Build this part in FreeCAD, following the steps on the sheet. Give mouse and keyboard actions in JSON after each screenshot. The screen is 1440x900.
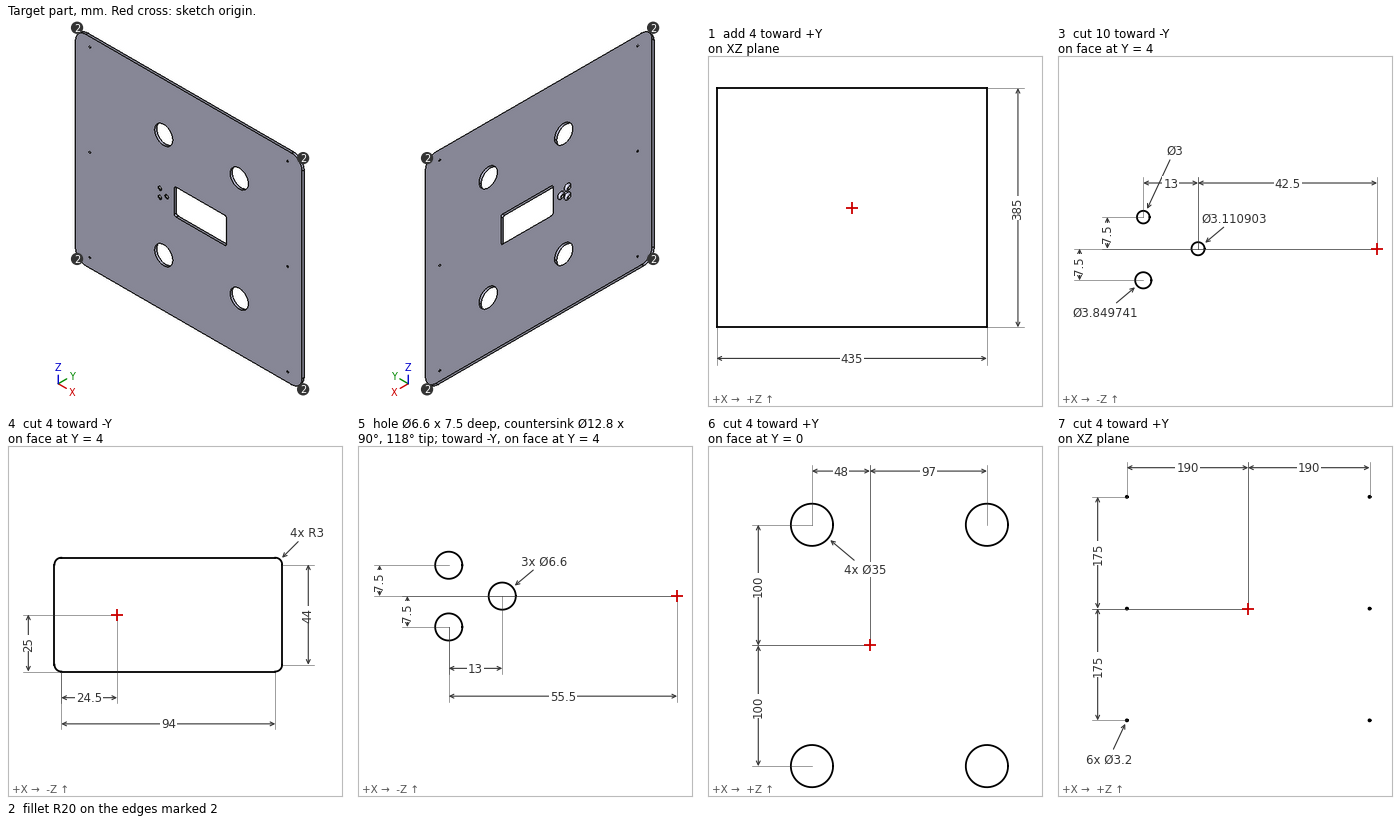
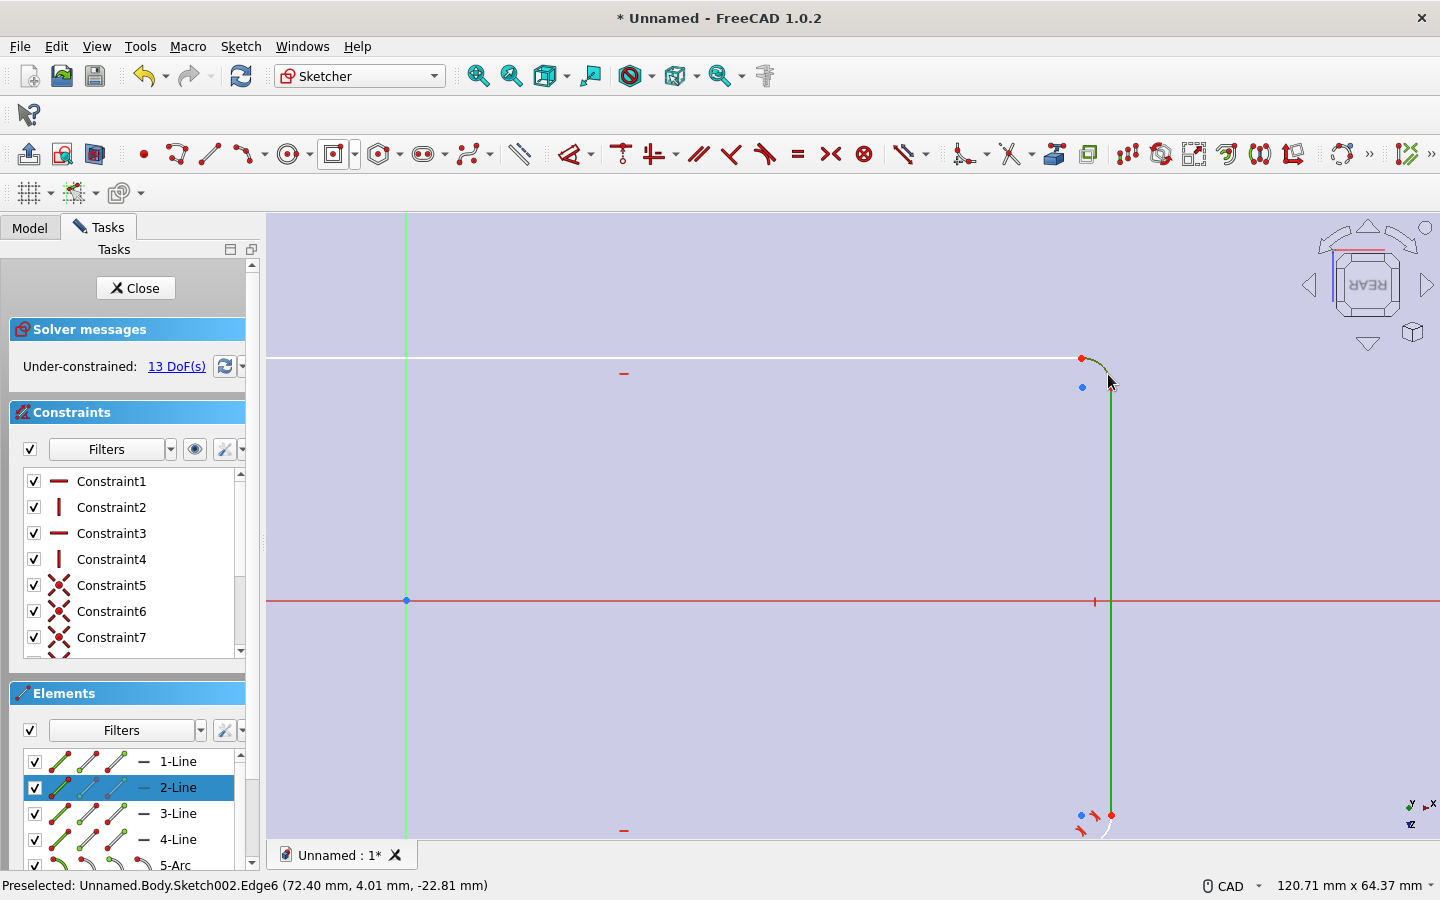
{"action": "left_click", "coordinate": [765, 154]}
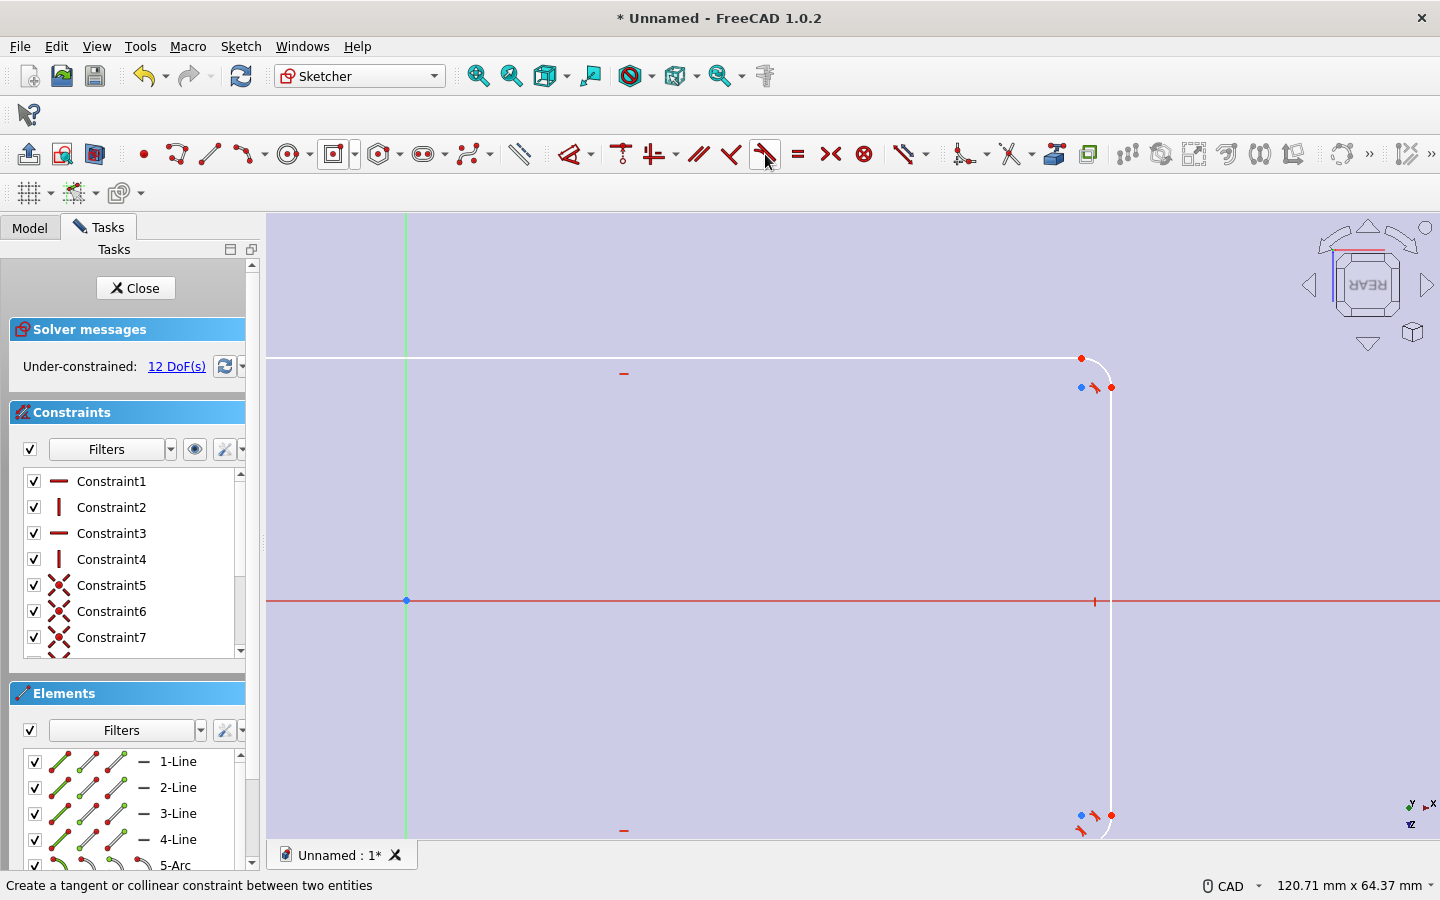
{"action": "left_click", "coordinate": [807, 358]}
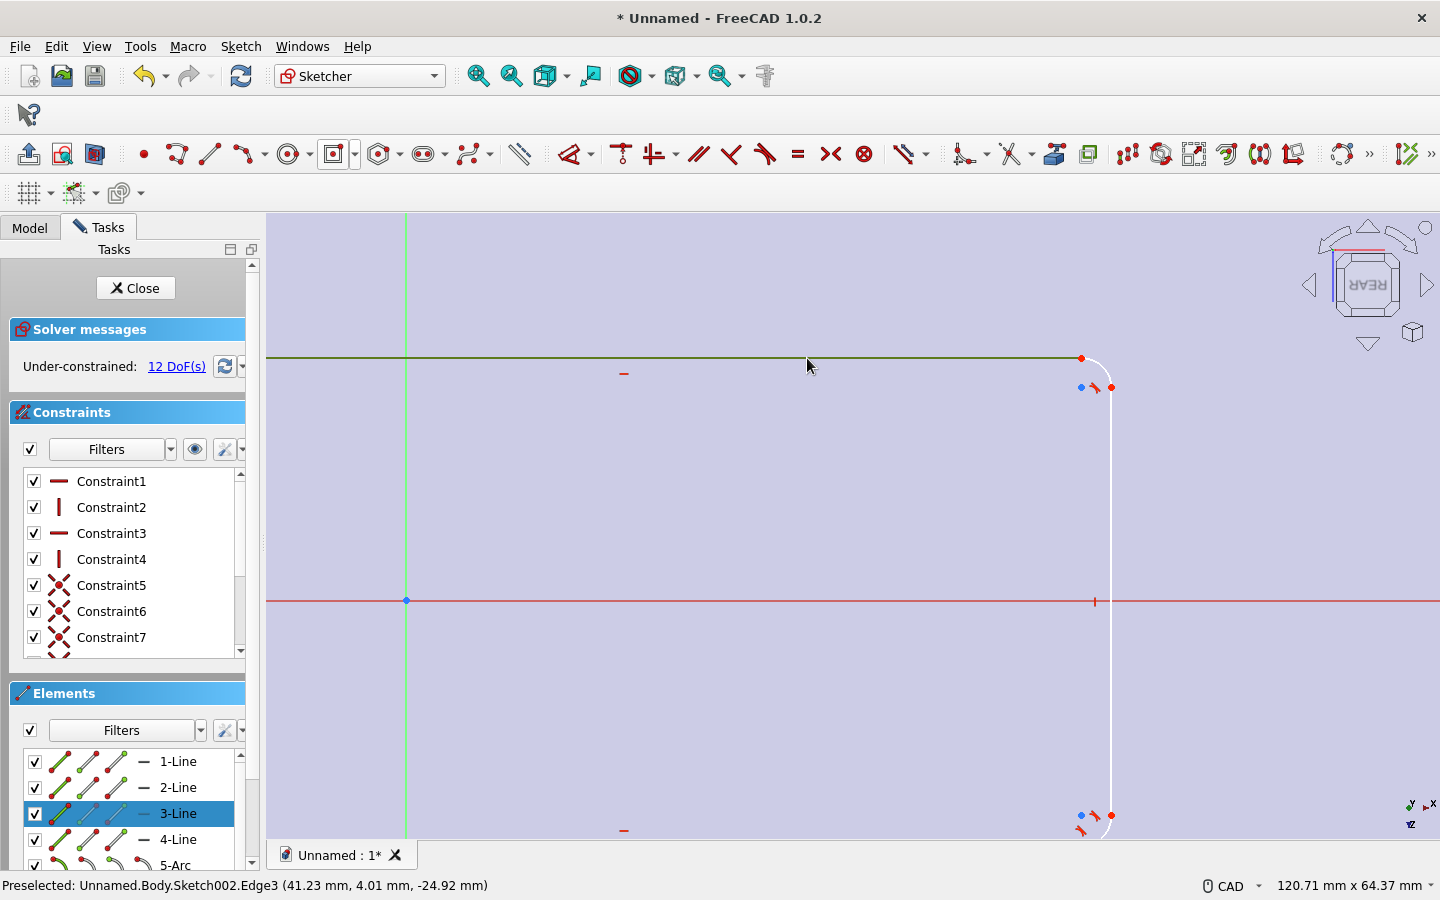
{"action": "left_click", "coordinate": [1108, 374]}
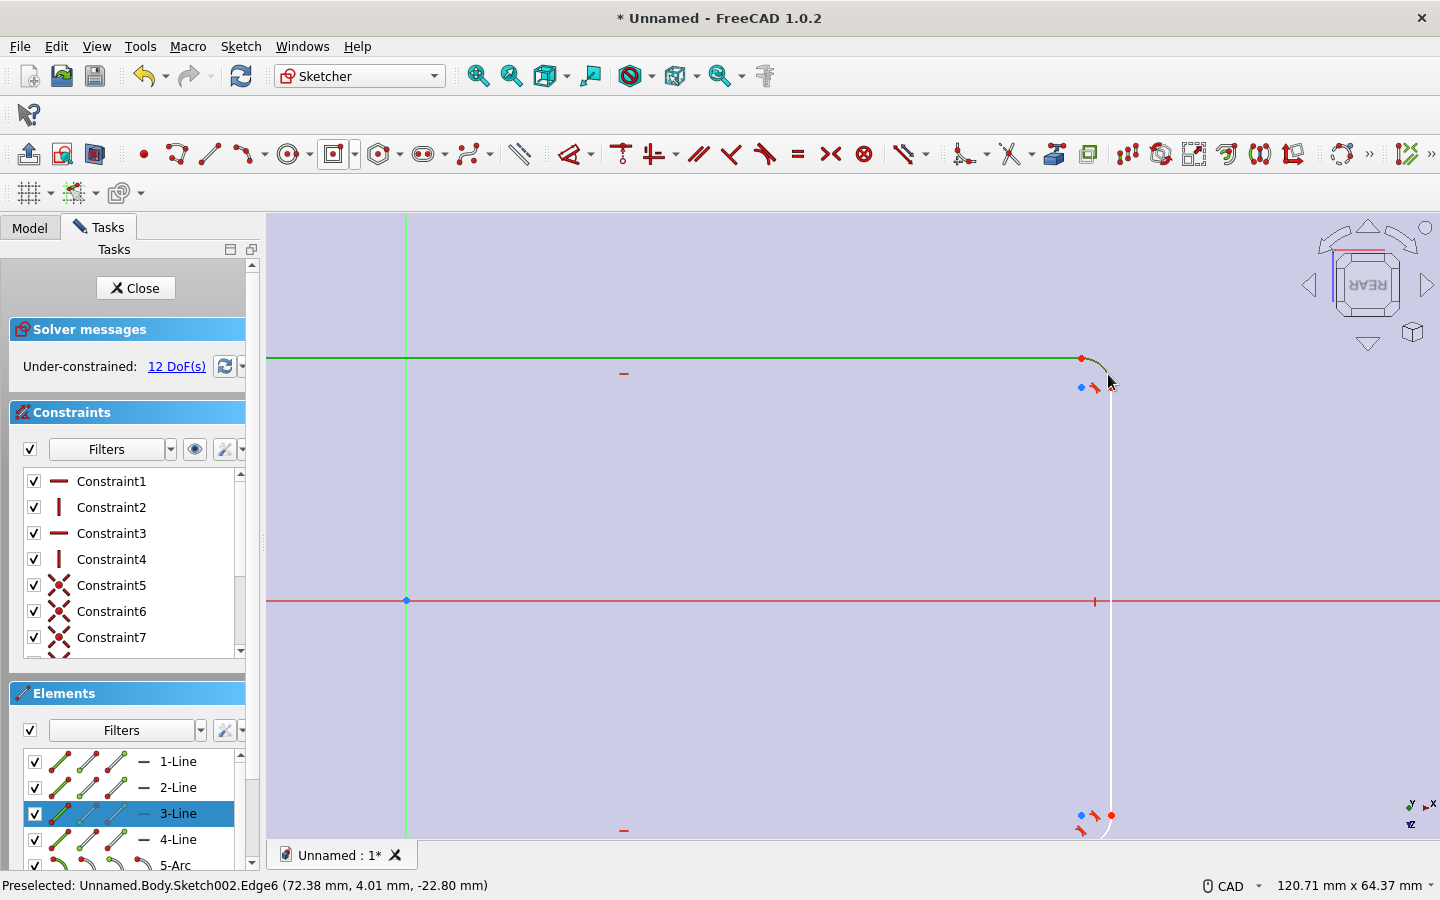
{"action": "left_click", "coordinate": [765, 154]}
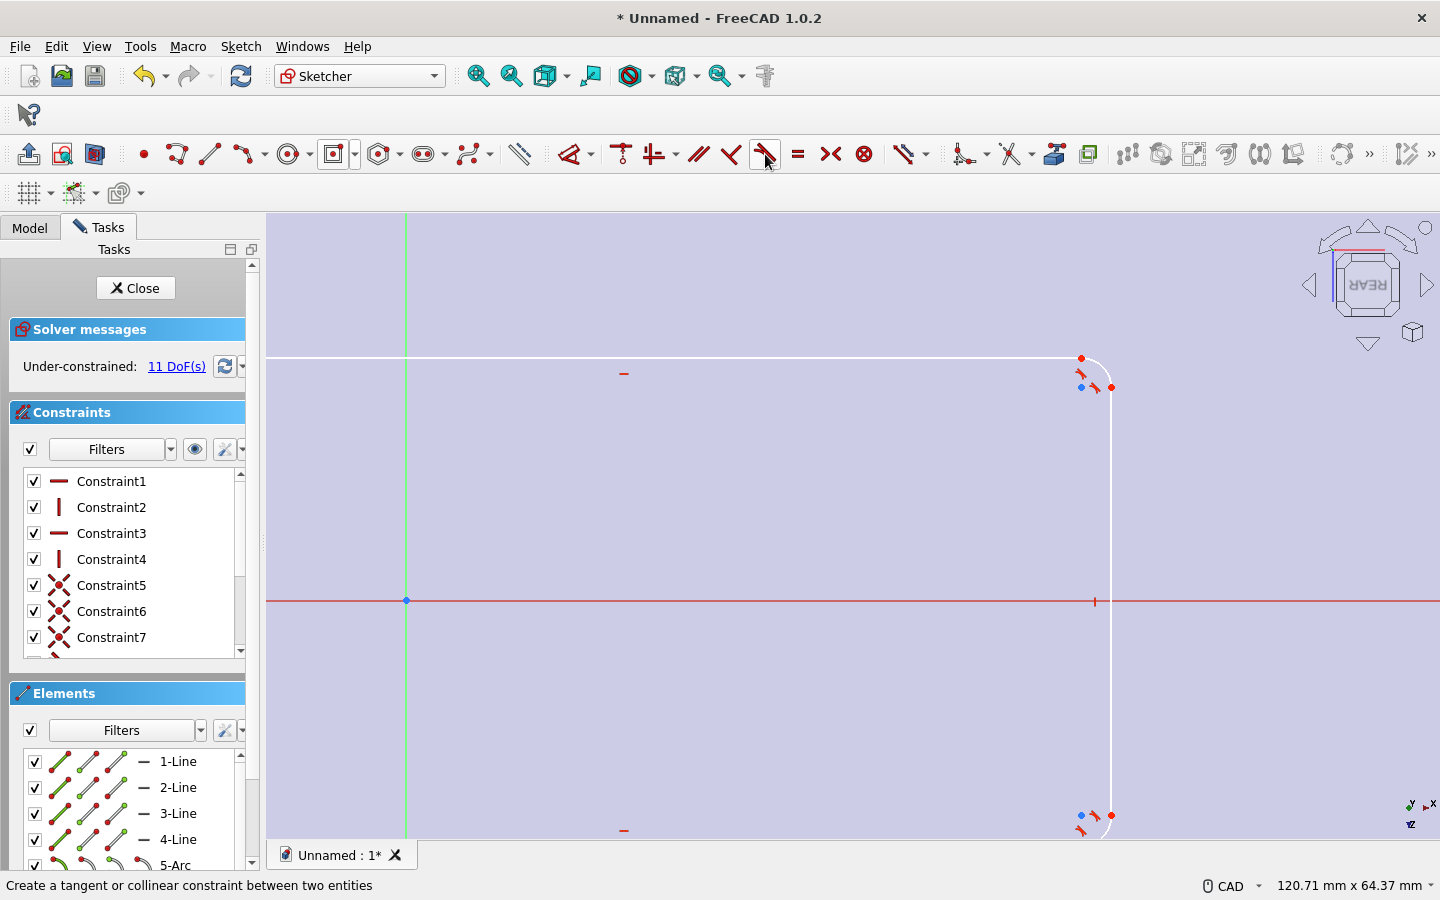
{"action": "left_click", "coordinate": [807, 358]}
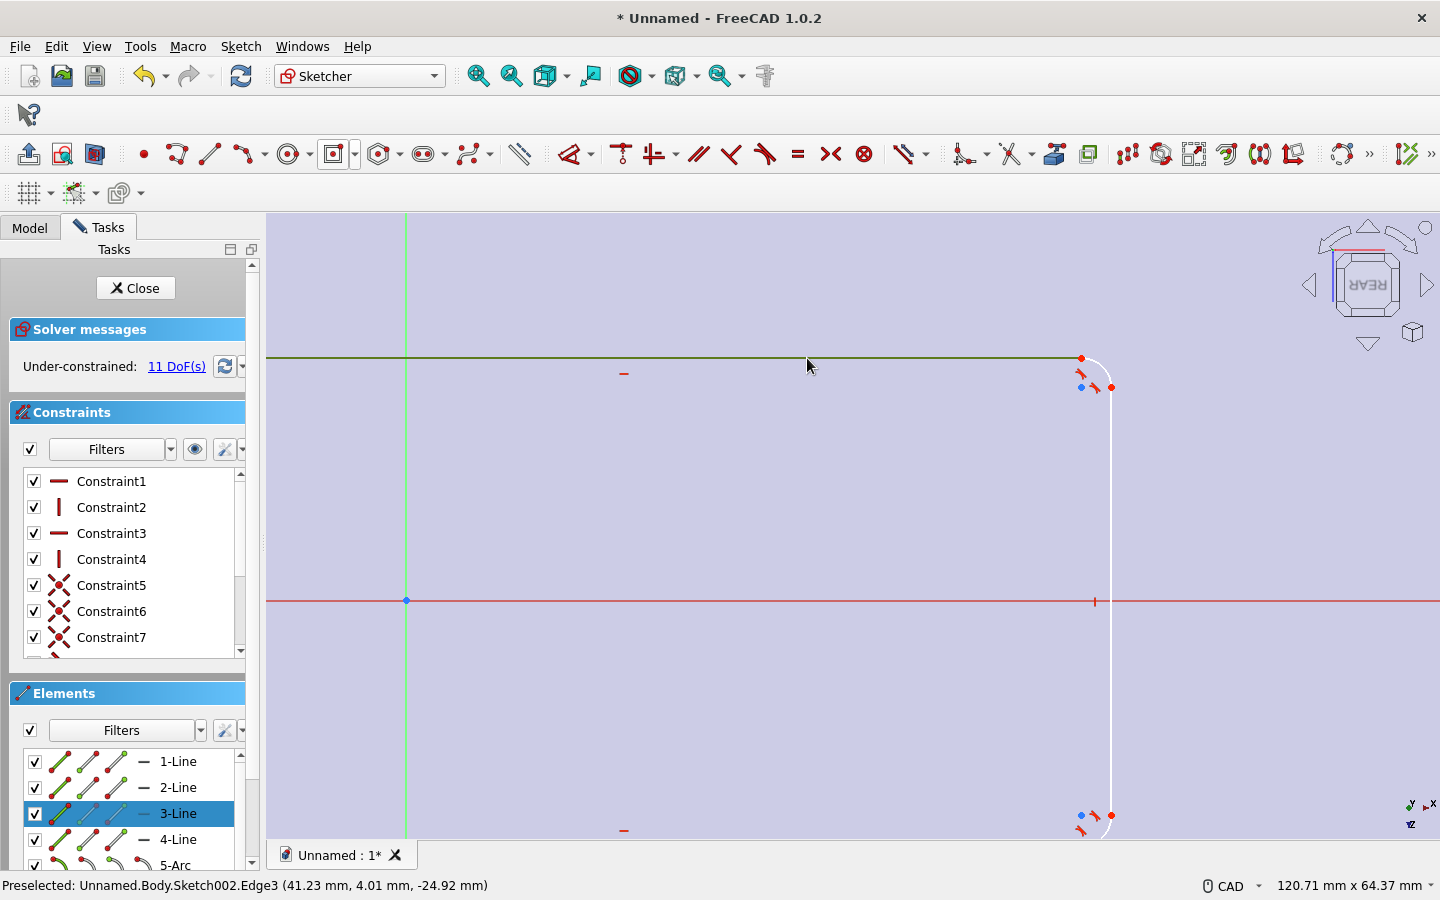
{"action": "scroll", "coordinate": [1109, 374], "scroll_direction": "down", "scroll_amount": 2}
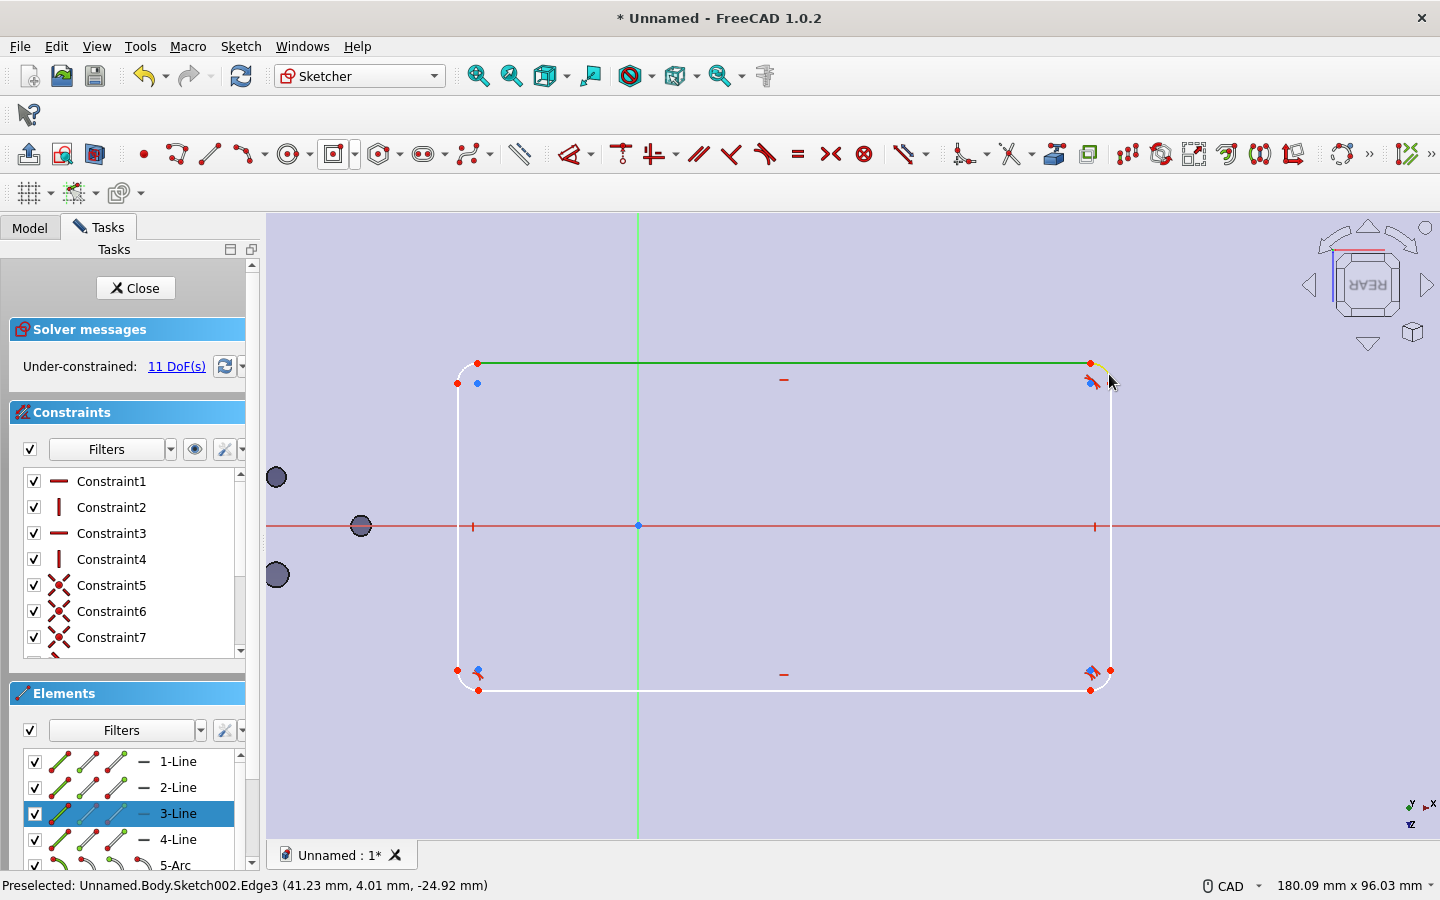
{"action": "scroll", "coordinate": [469, 366], "scroll_direction": "up", "scroll_amount": 2}